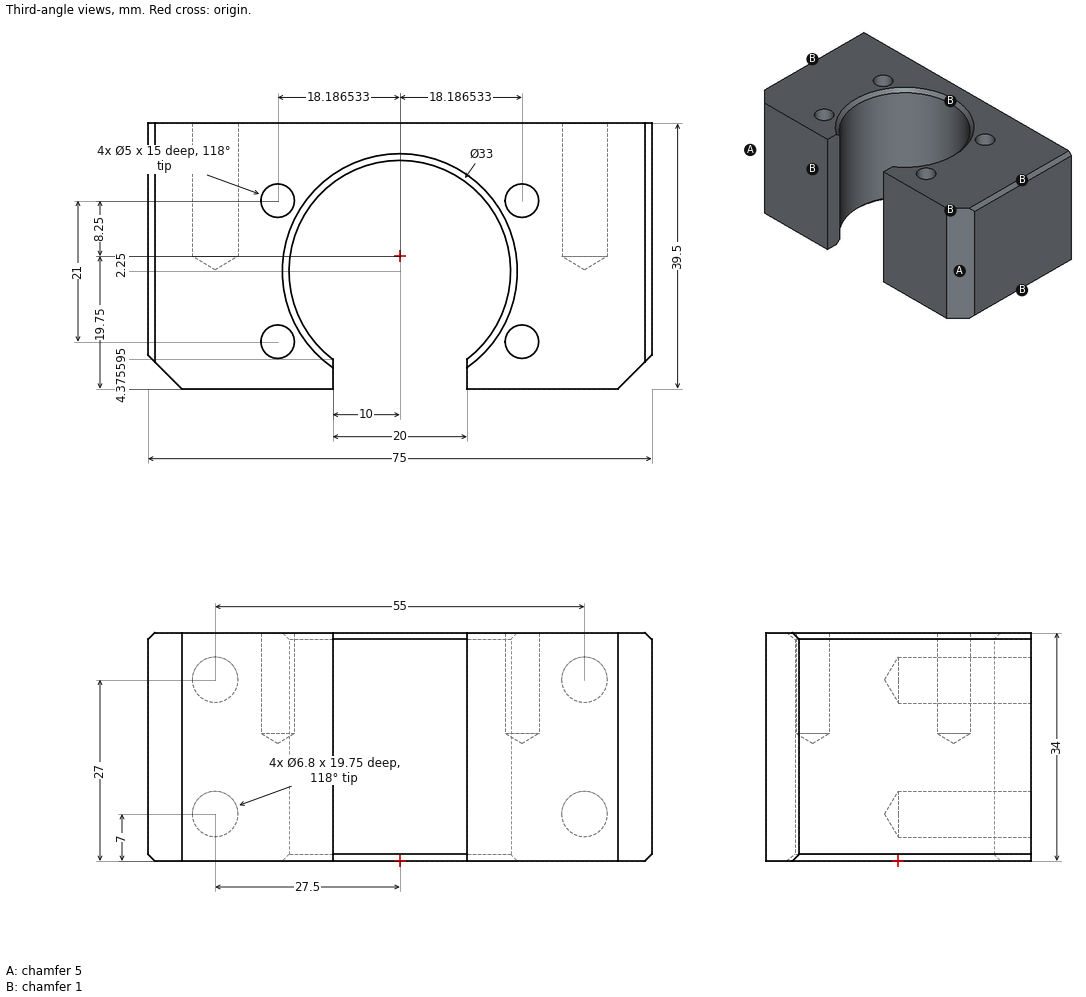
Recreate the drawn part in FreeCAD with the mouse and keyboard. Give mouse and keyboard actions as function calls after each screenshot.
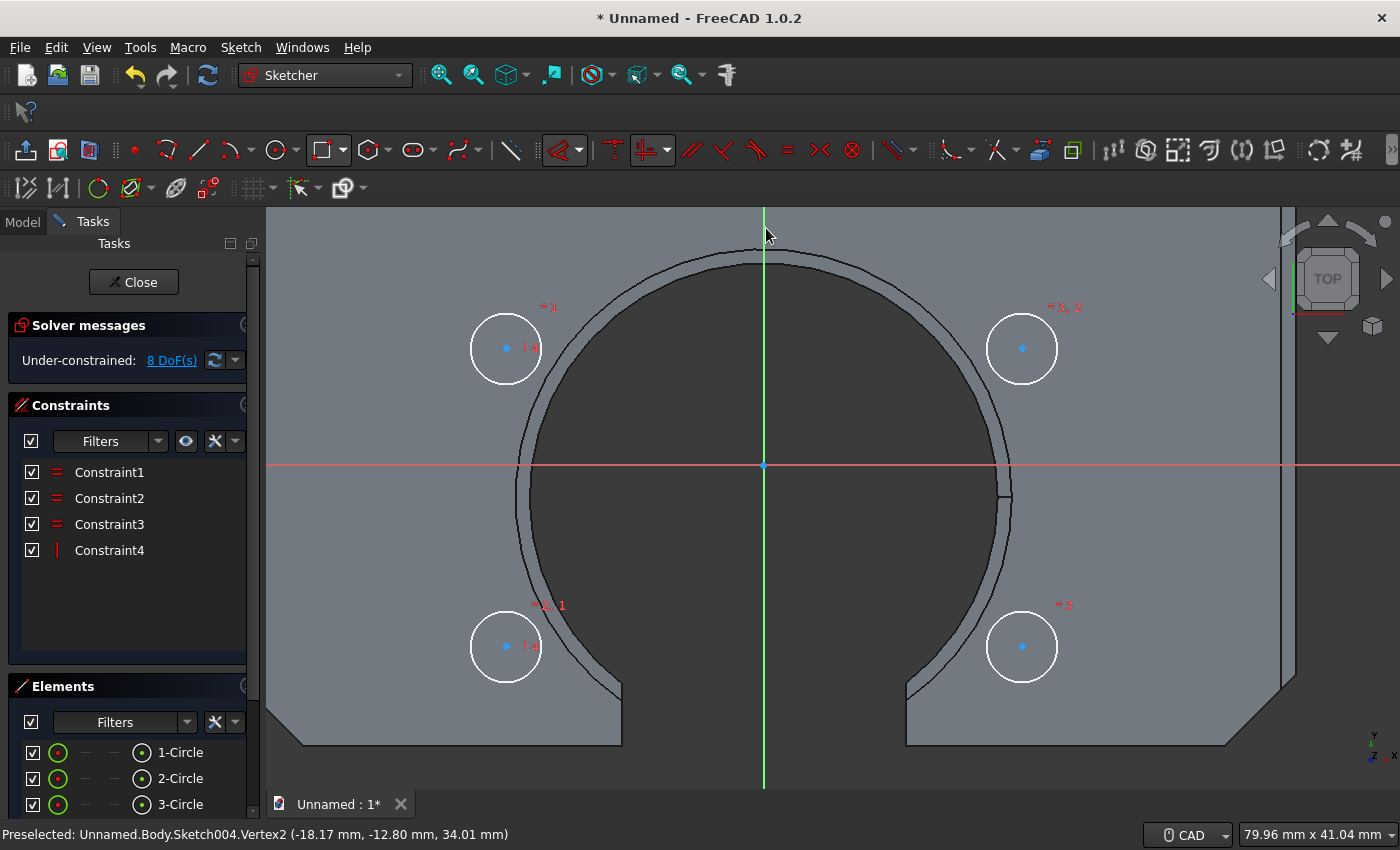
click(506, 349)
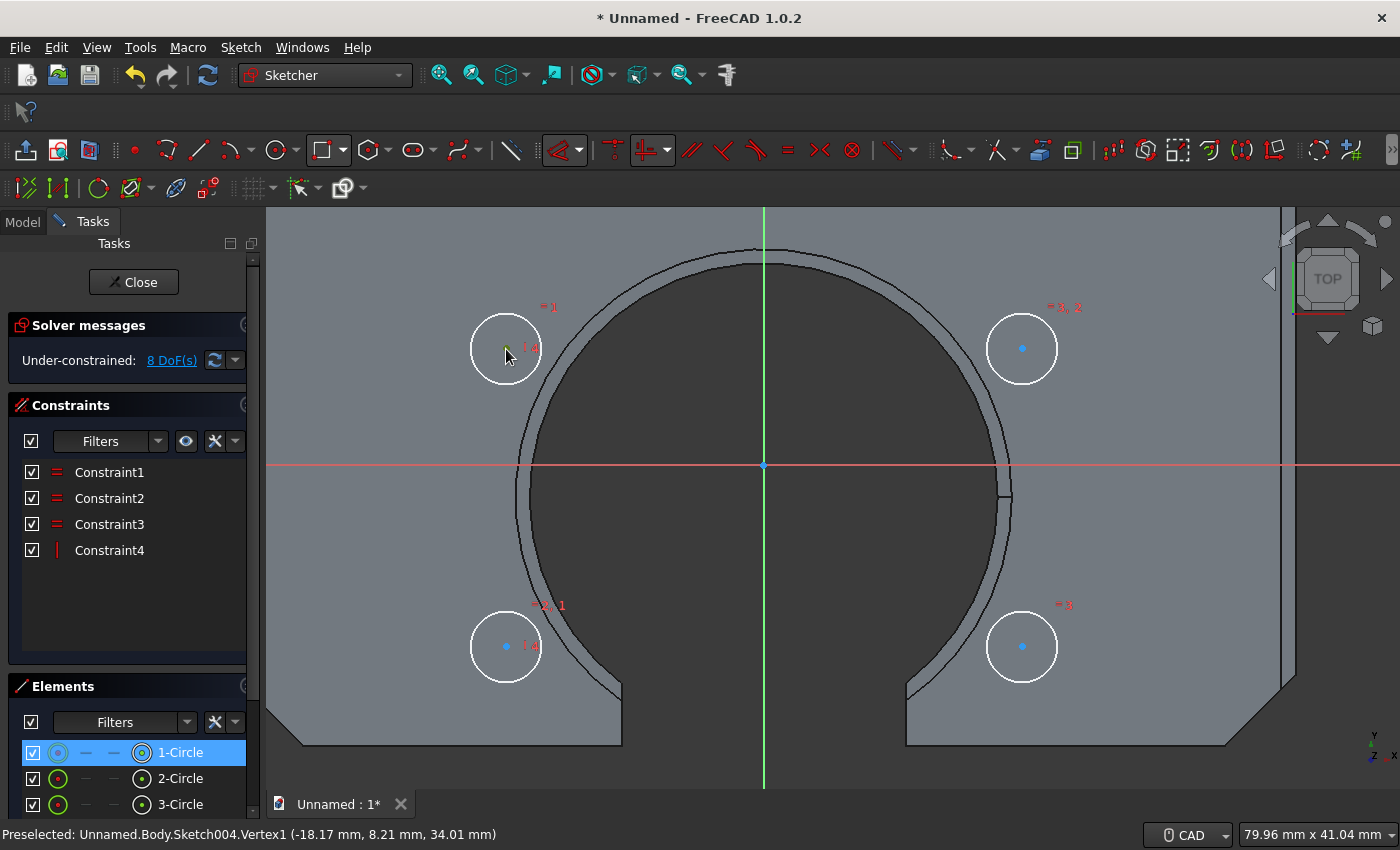
click(1022, 349)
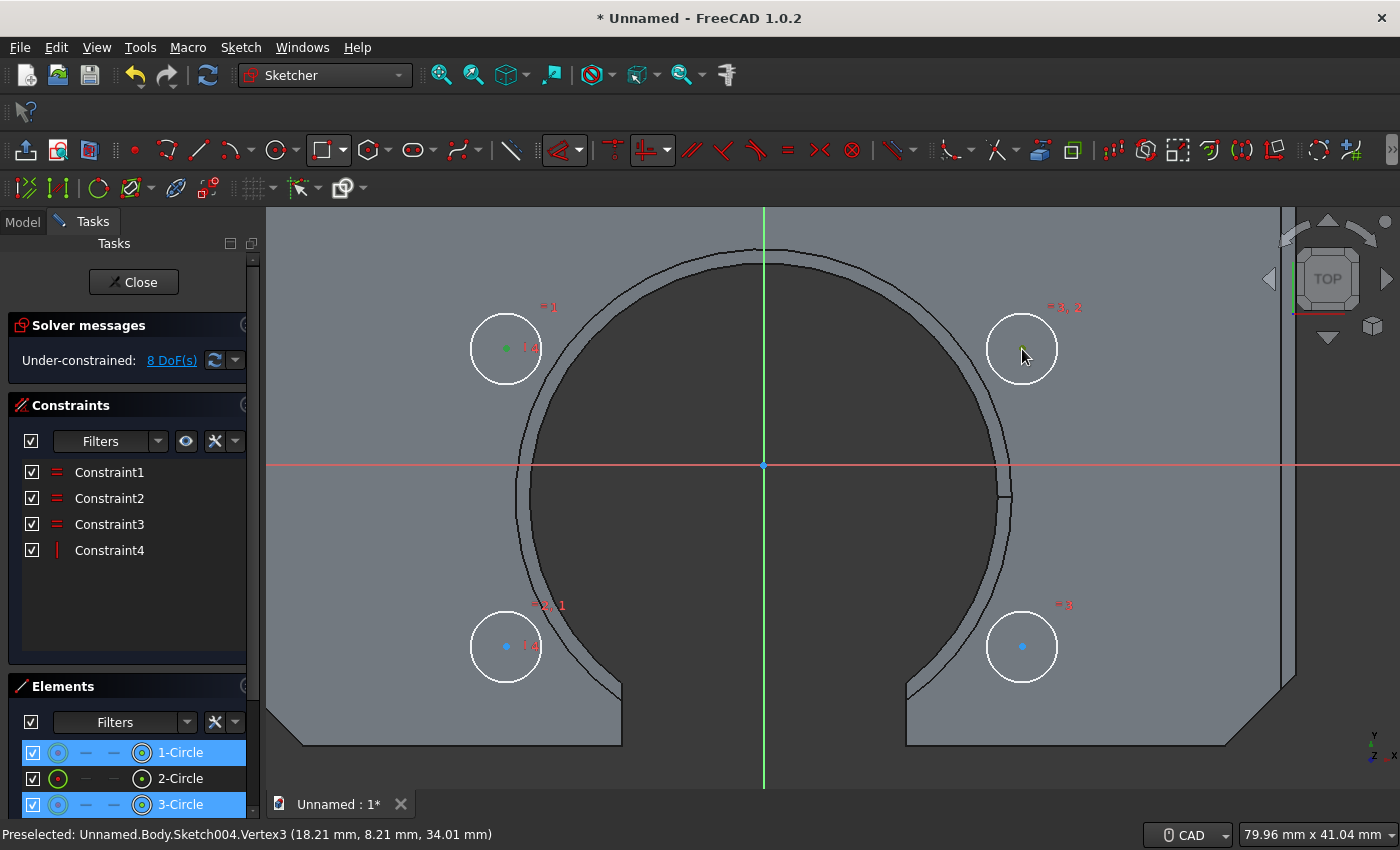
click(670, 150)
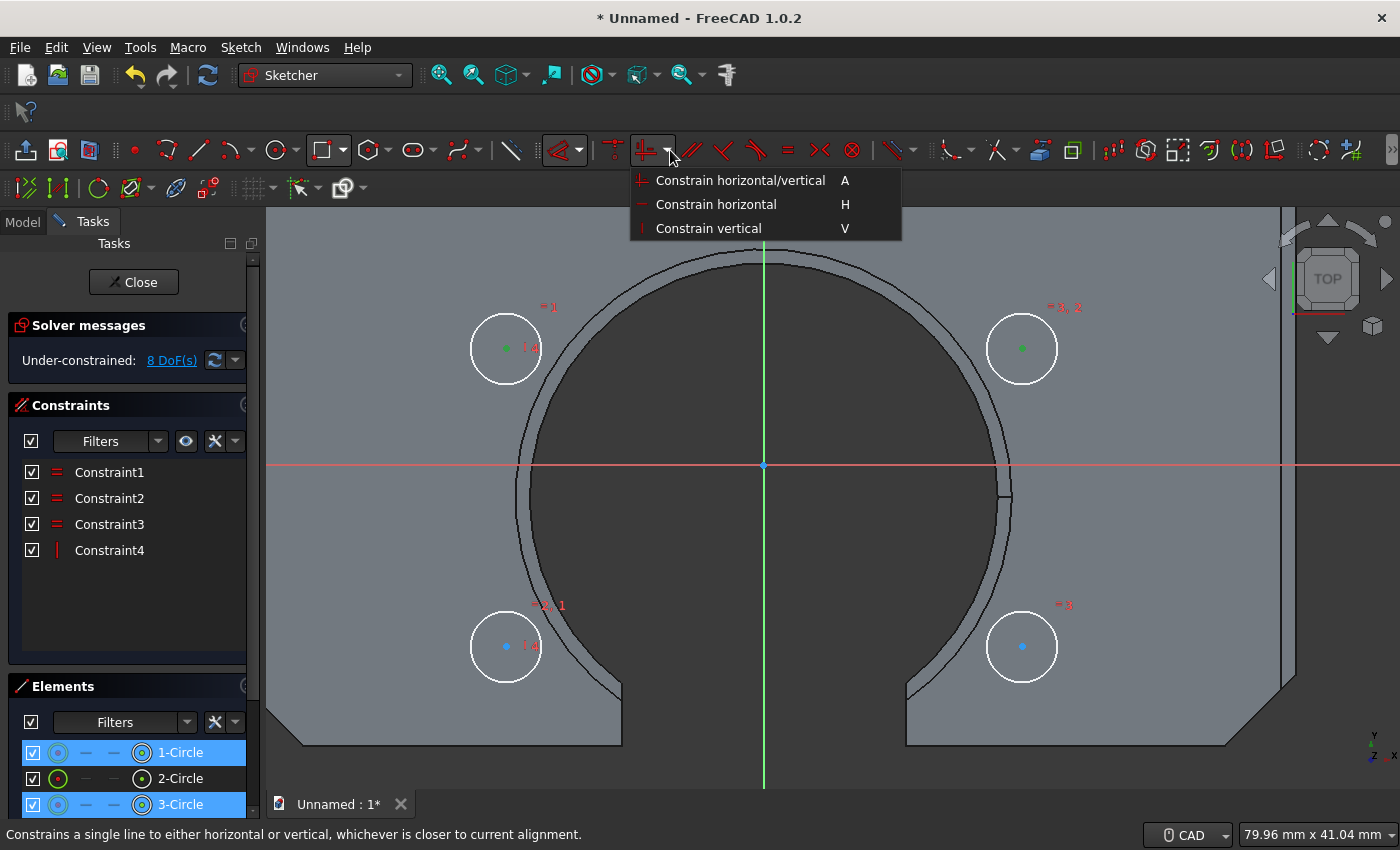
click(766, 204)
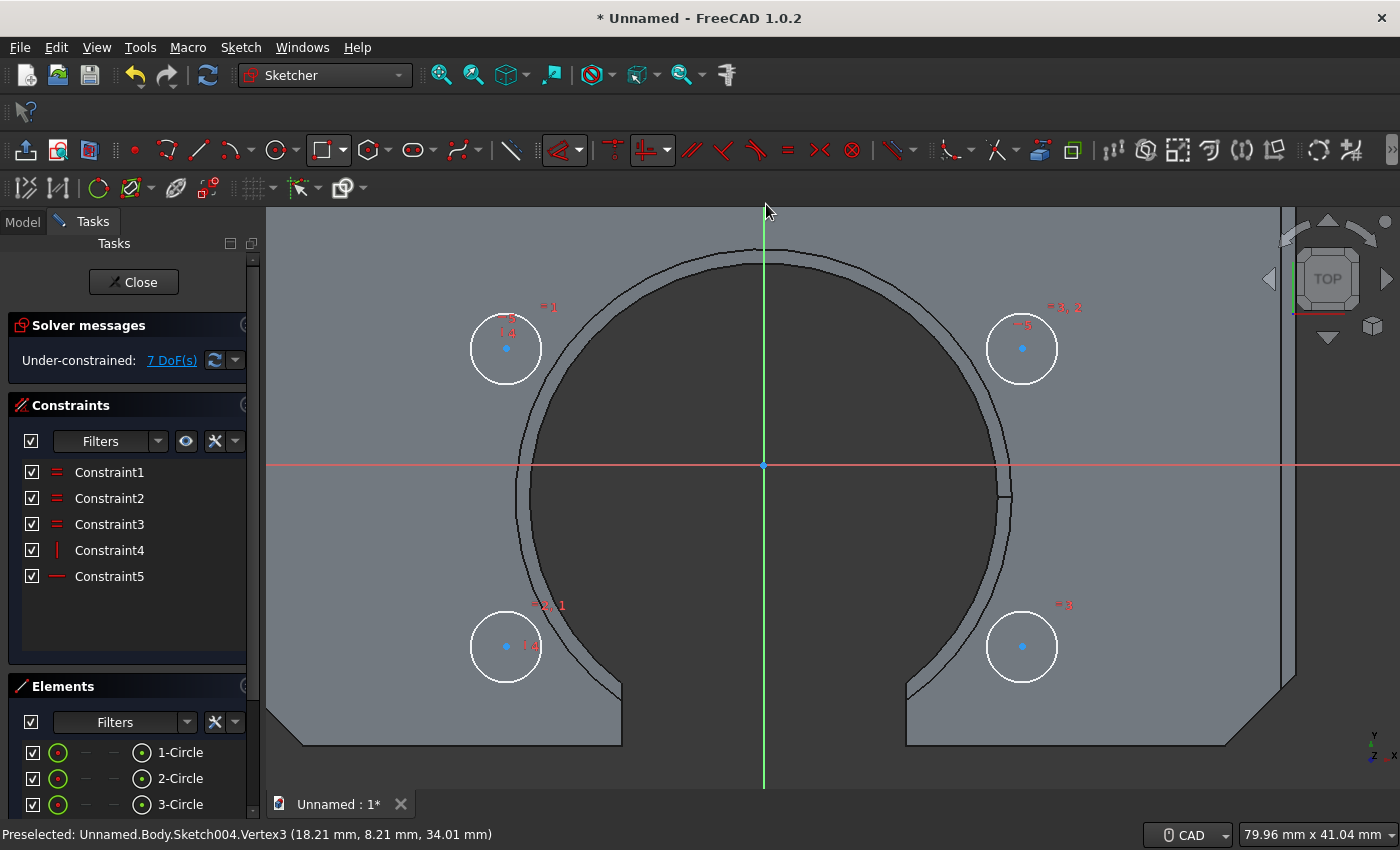
click(1022, 349)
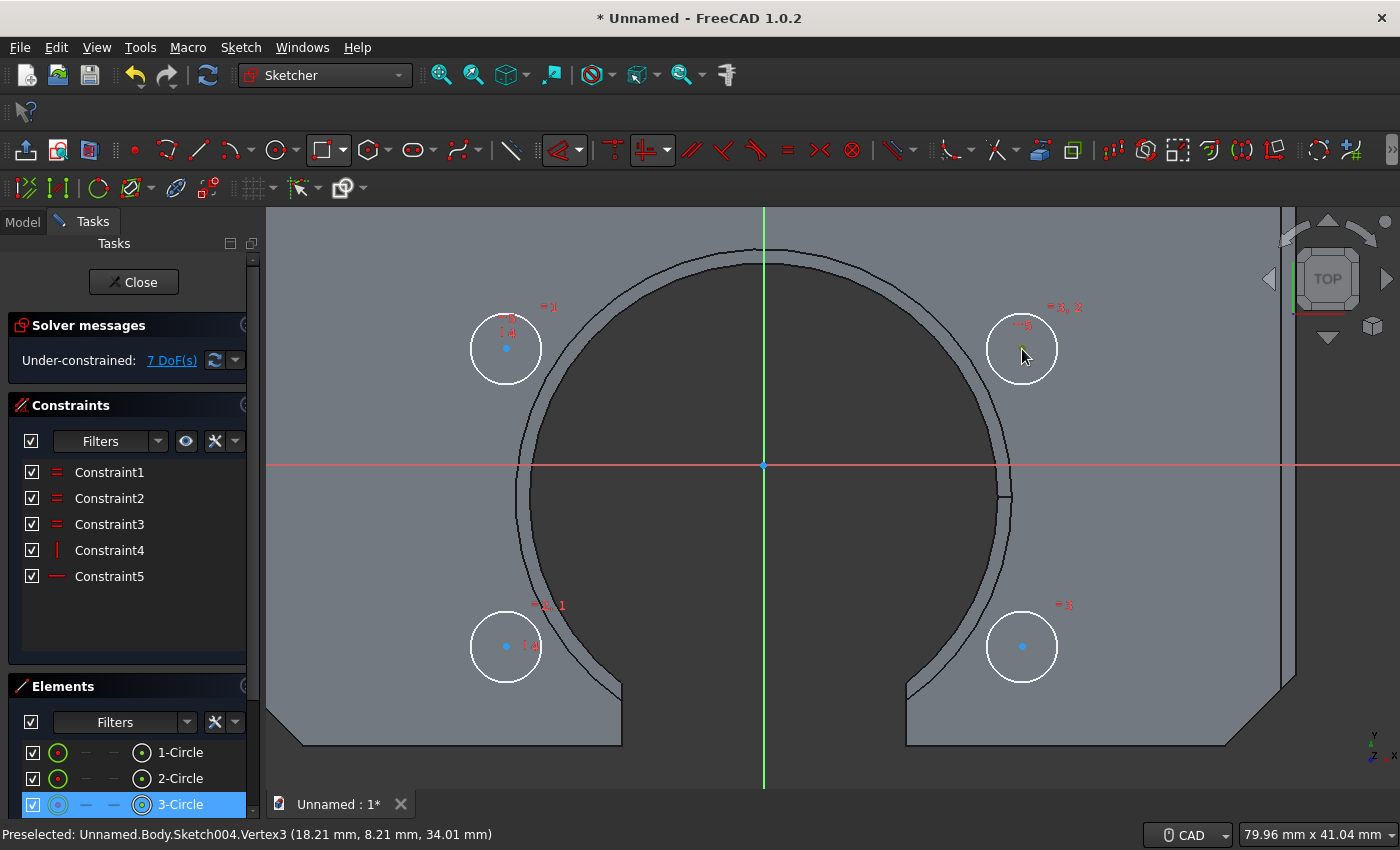
click(1022, 647)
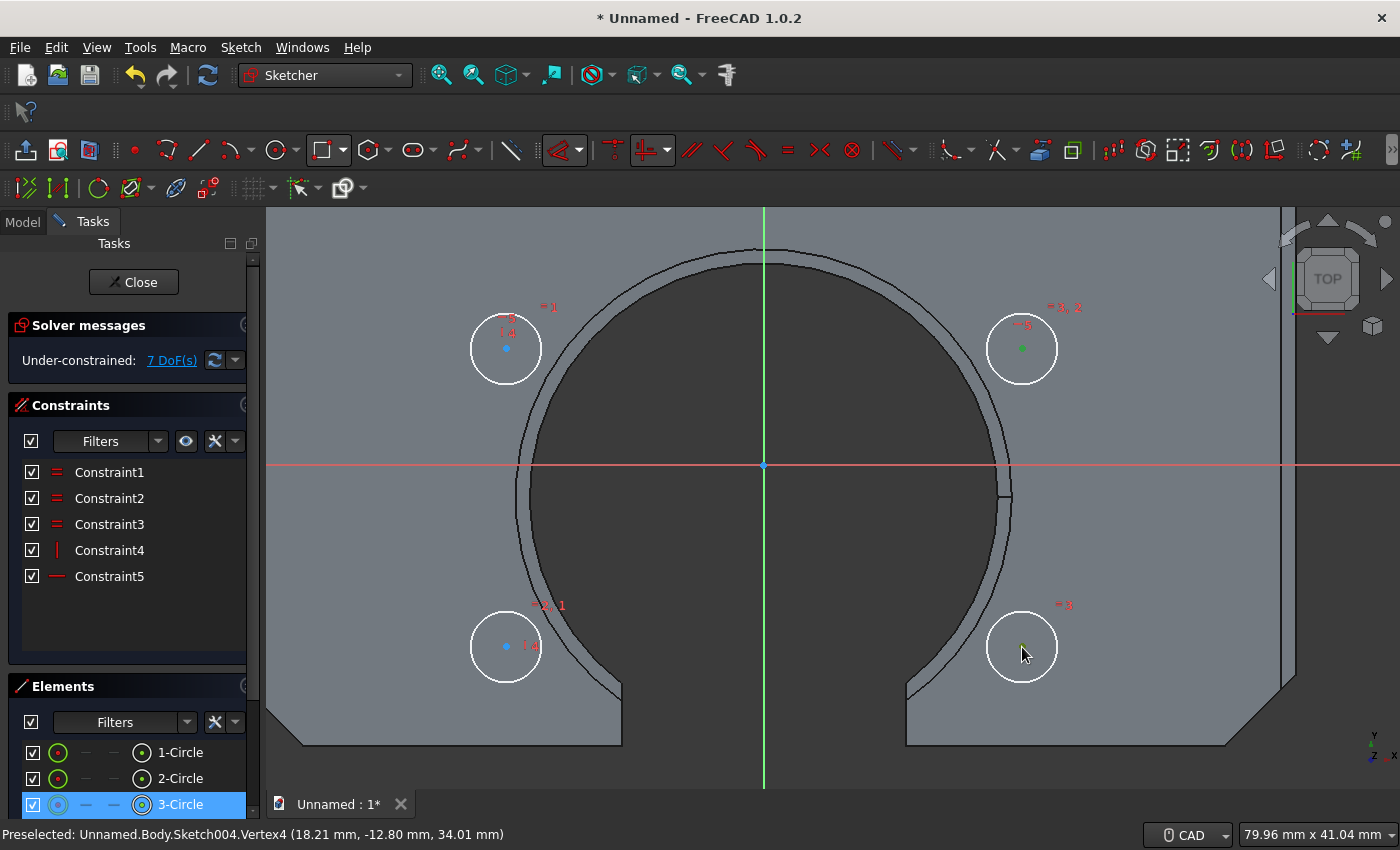
click(670, 150)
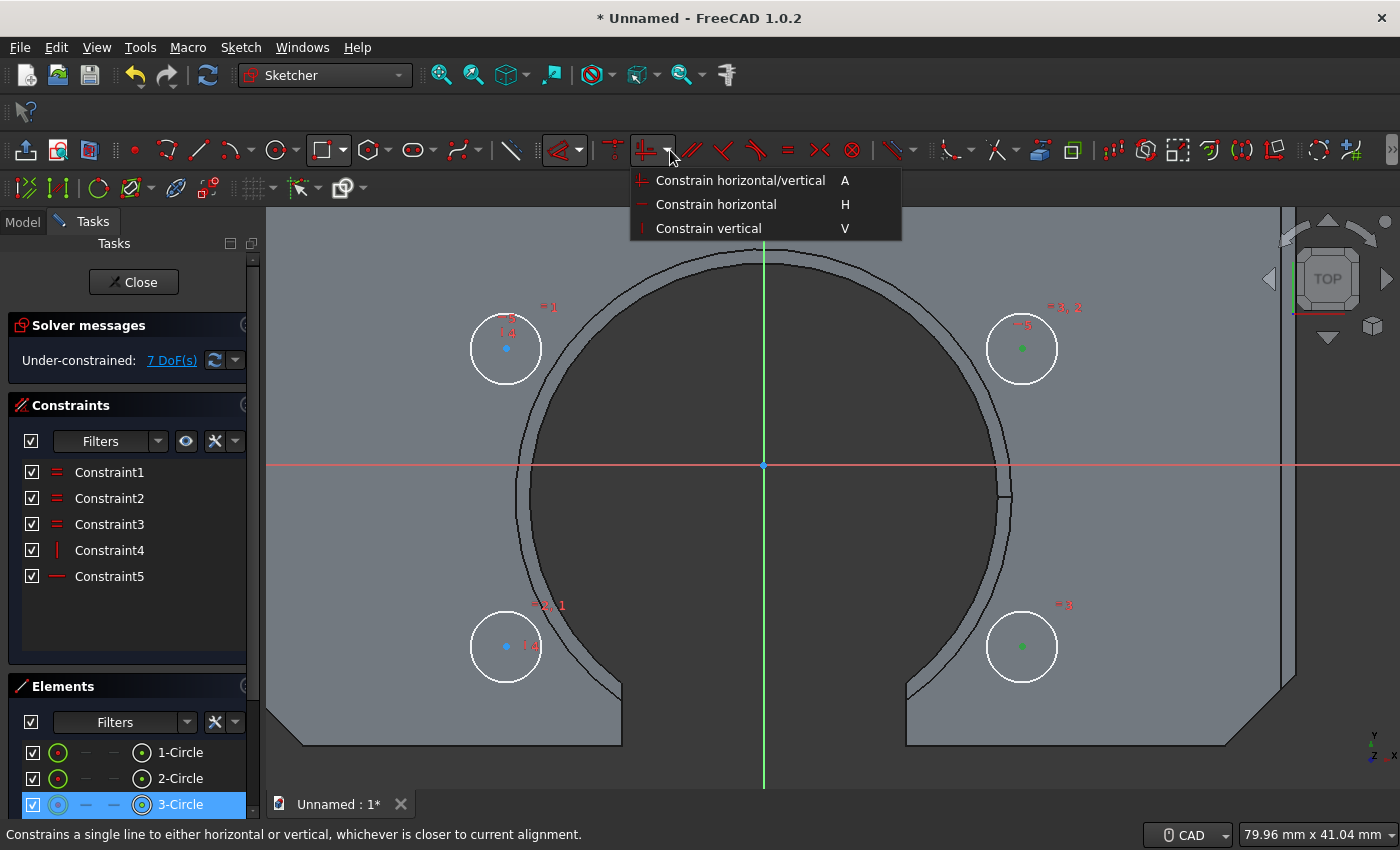
click(766, 228)